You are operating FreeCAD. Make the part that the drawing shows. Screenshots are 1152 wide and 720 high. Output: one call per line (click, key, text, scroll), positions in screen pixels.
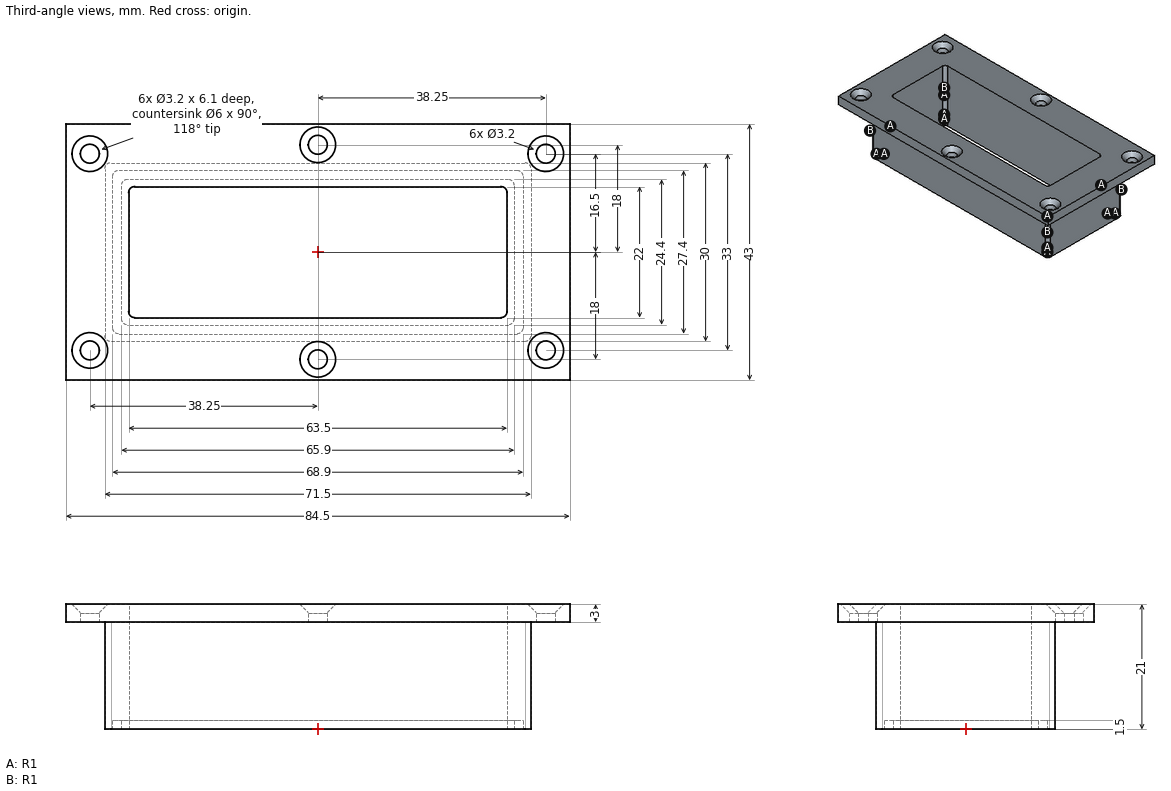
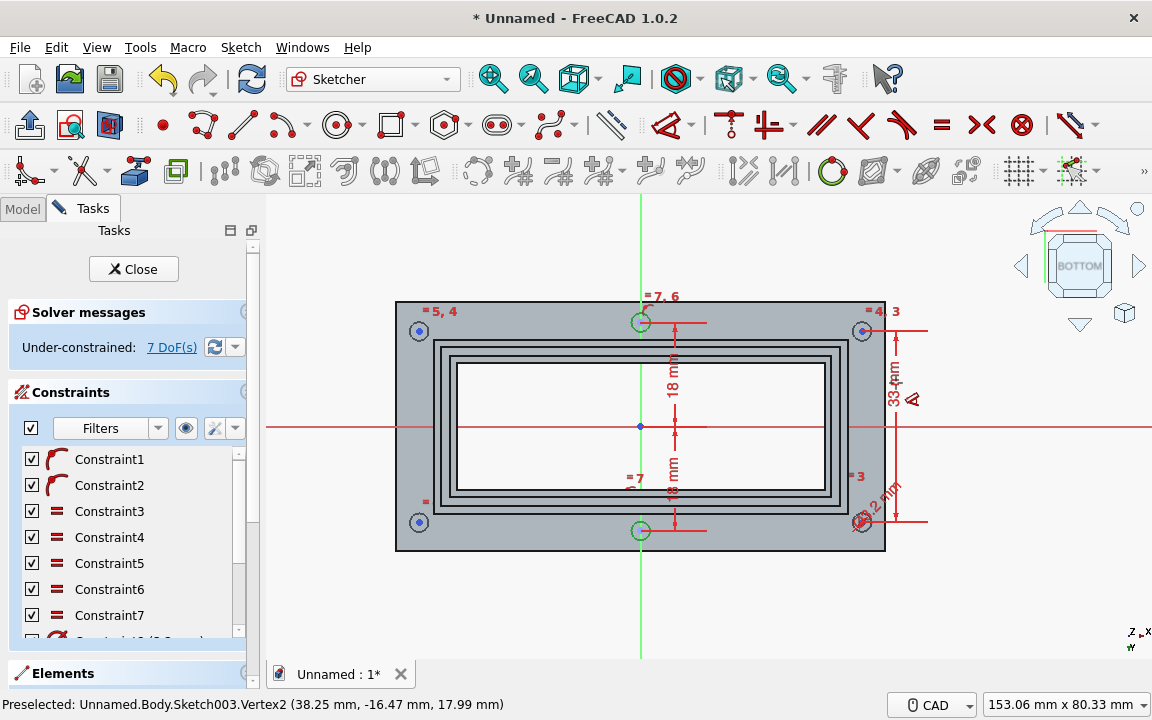
click(862, 522)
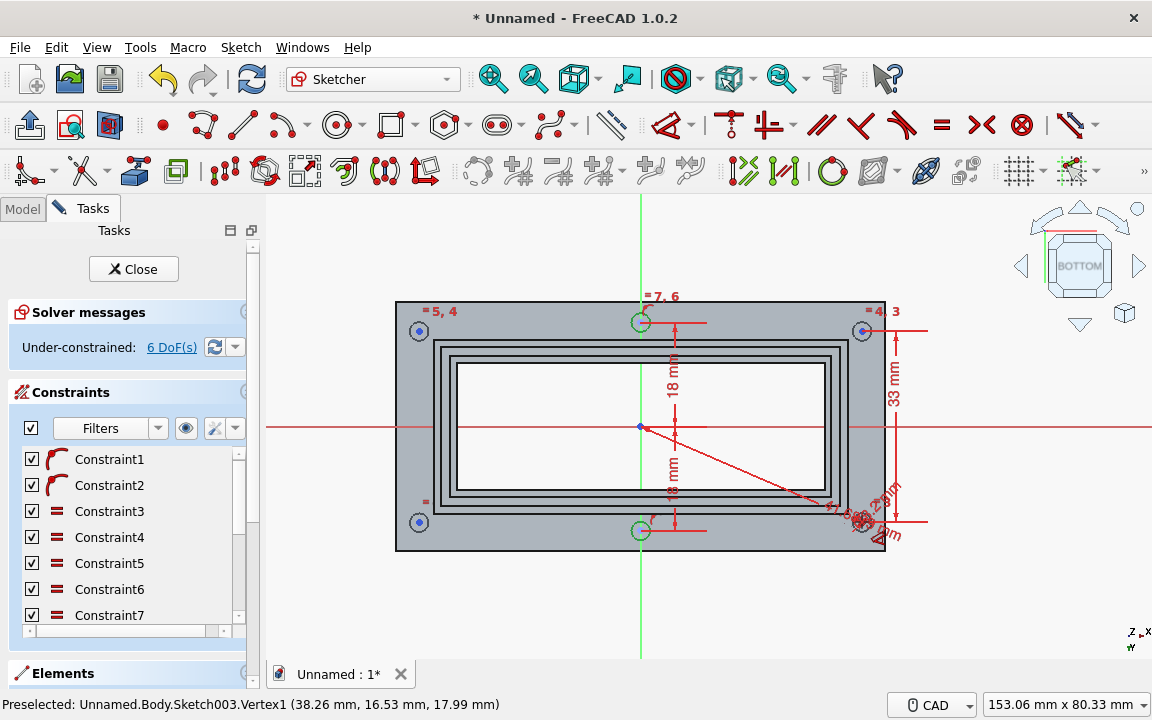
click(419, 331)
click(385, 383)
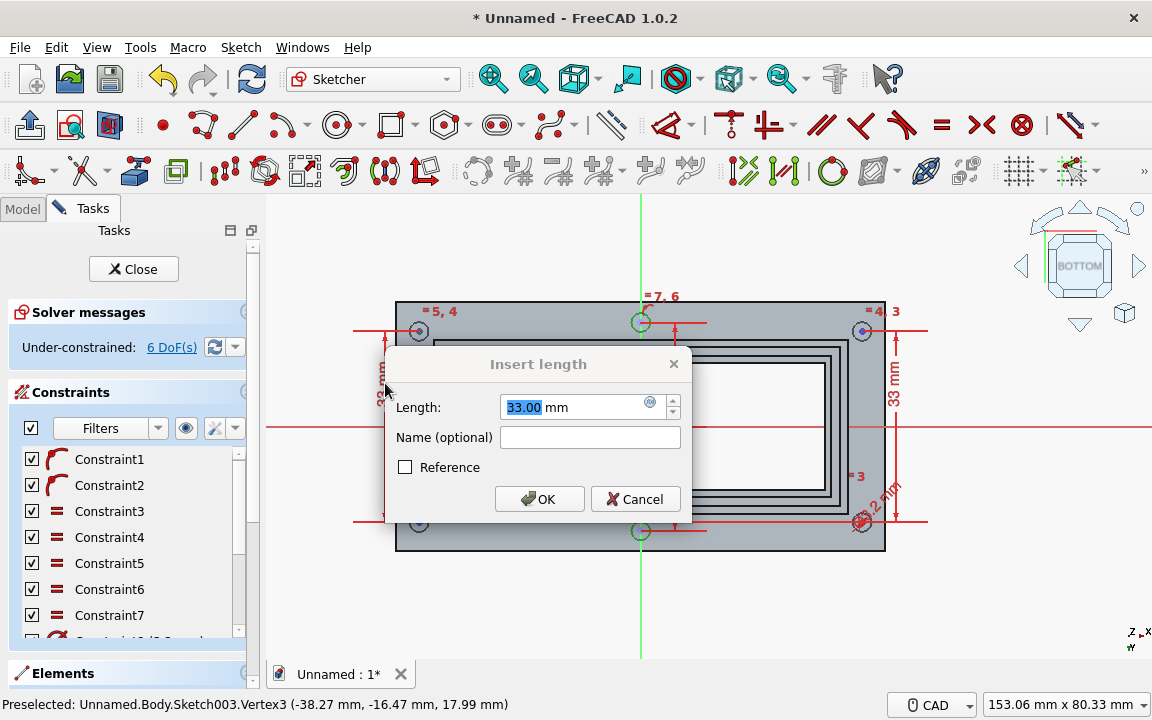
text(33)
key(Return)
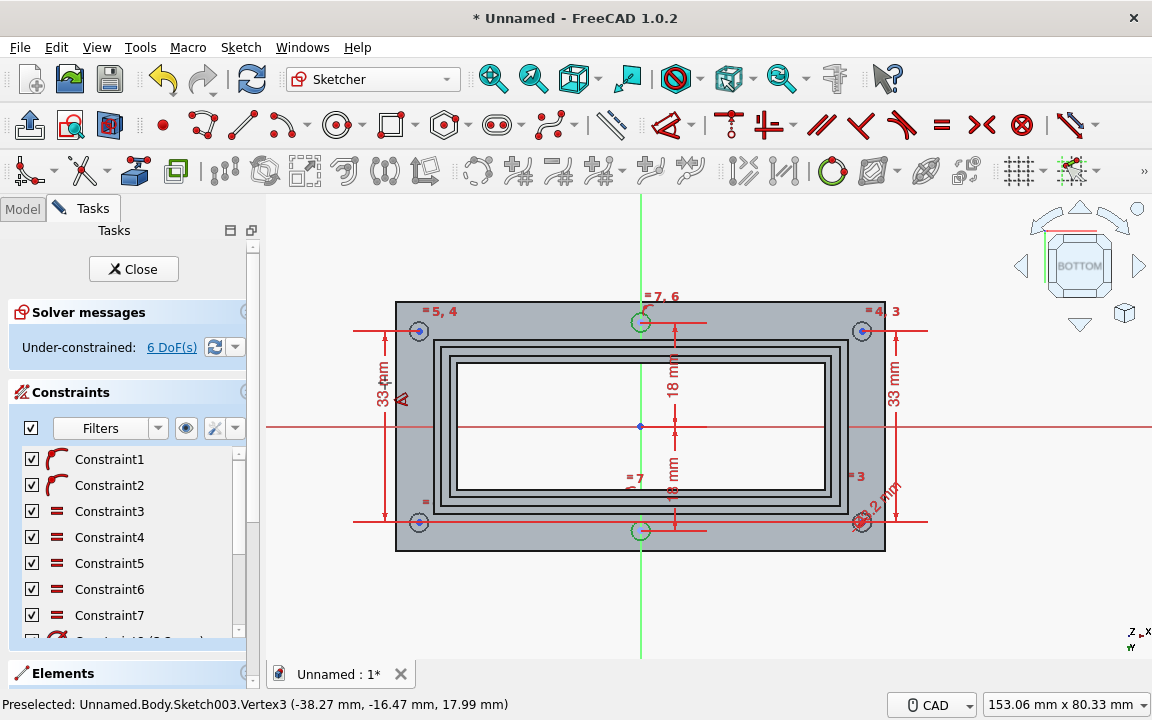
click(419, 331)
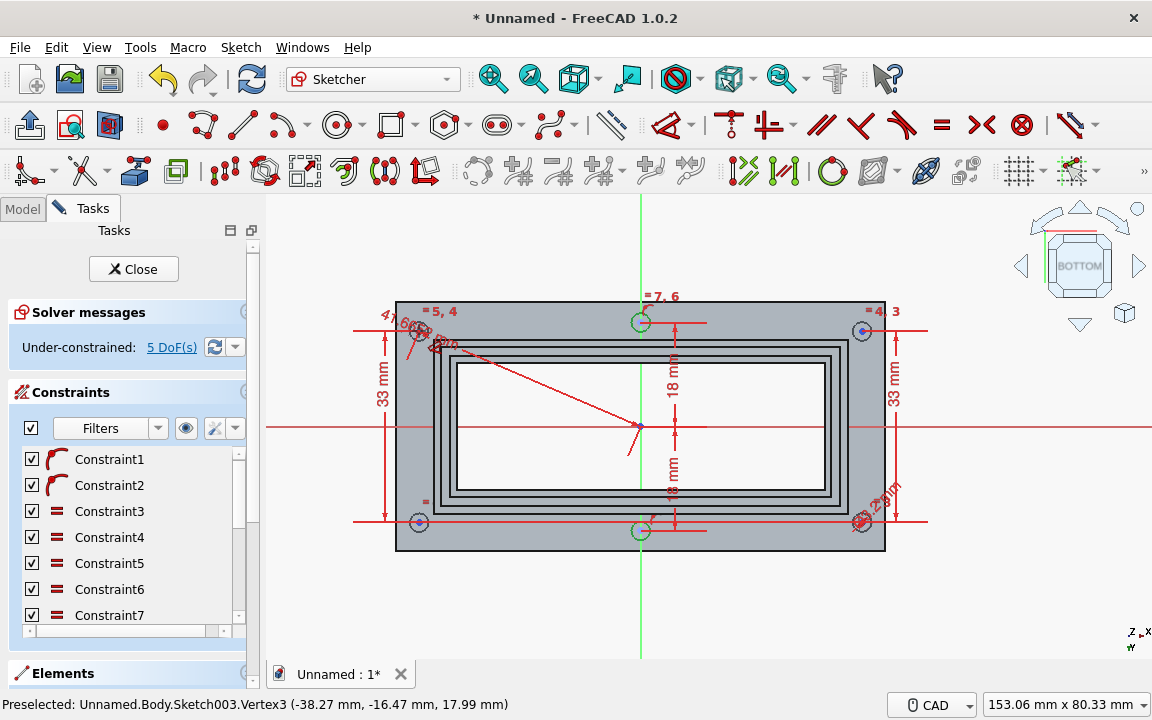
click(419, 523)
click(385, 471)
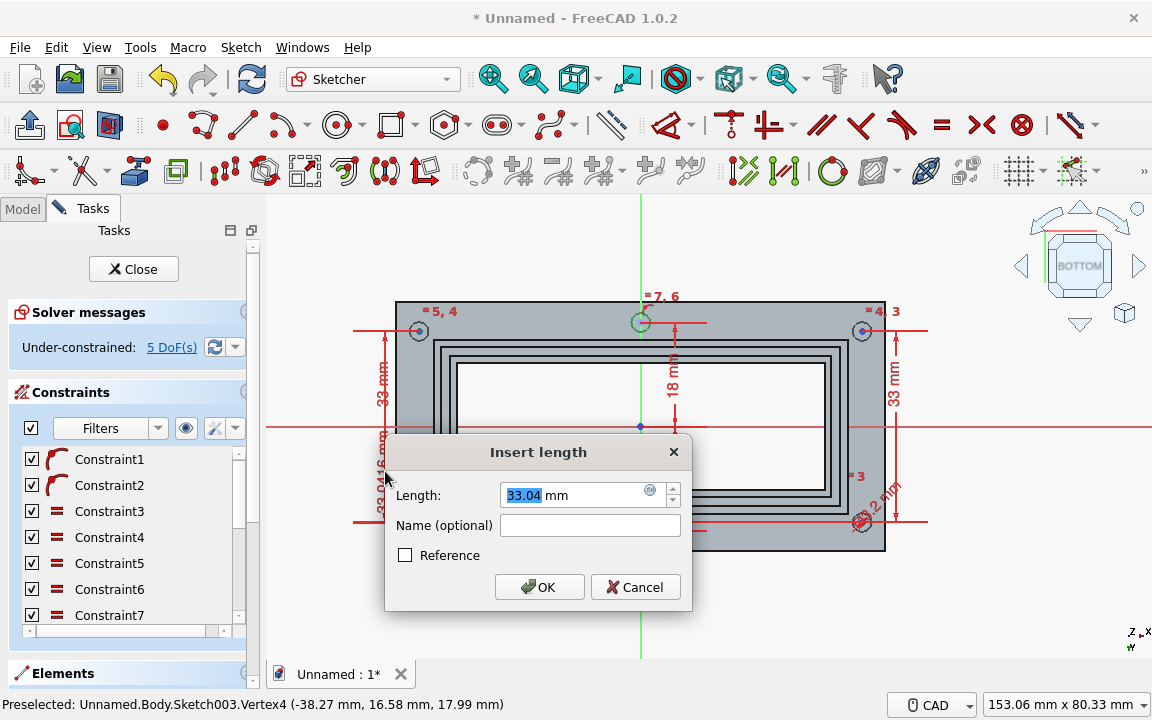
text(33)
key(Return)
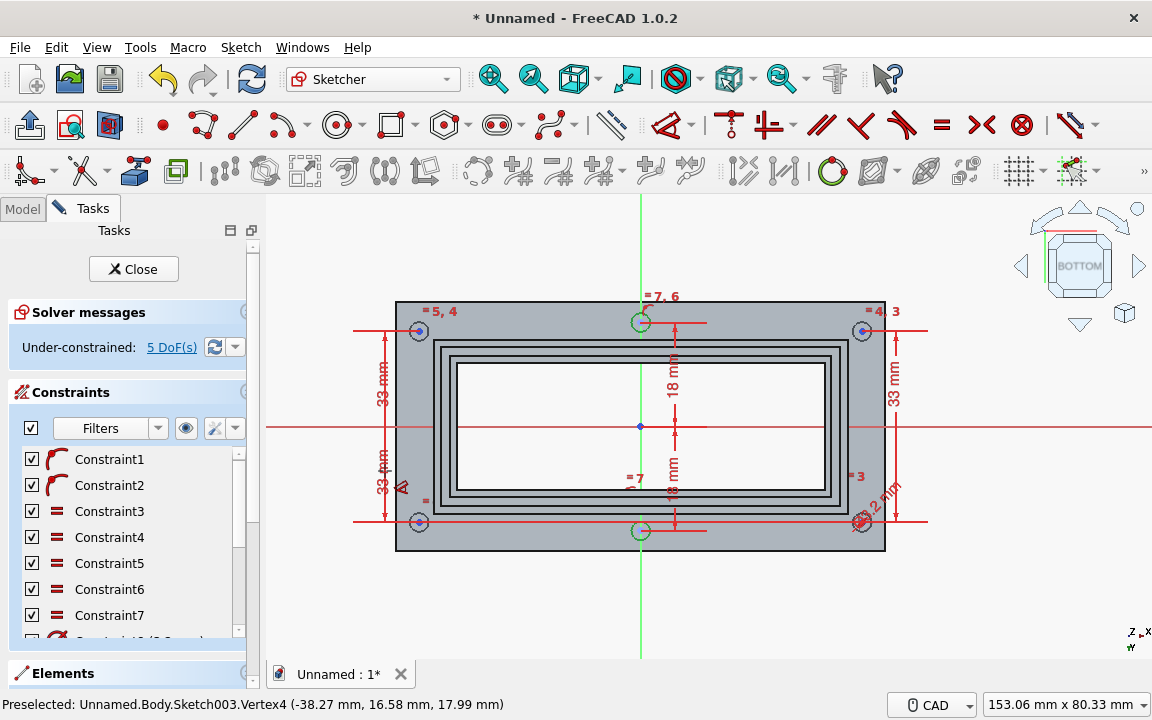
click(862, 522)
click(896, 475)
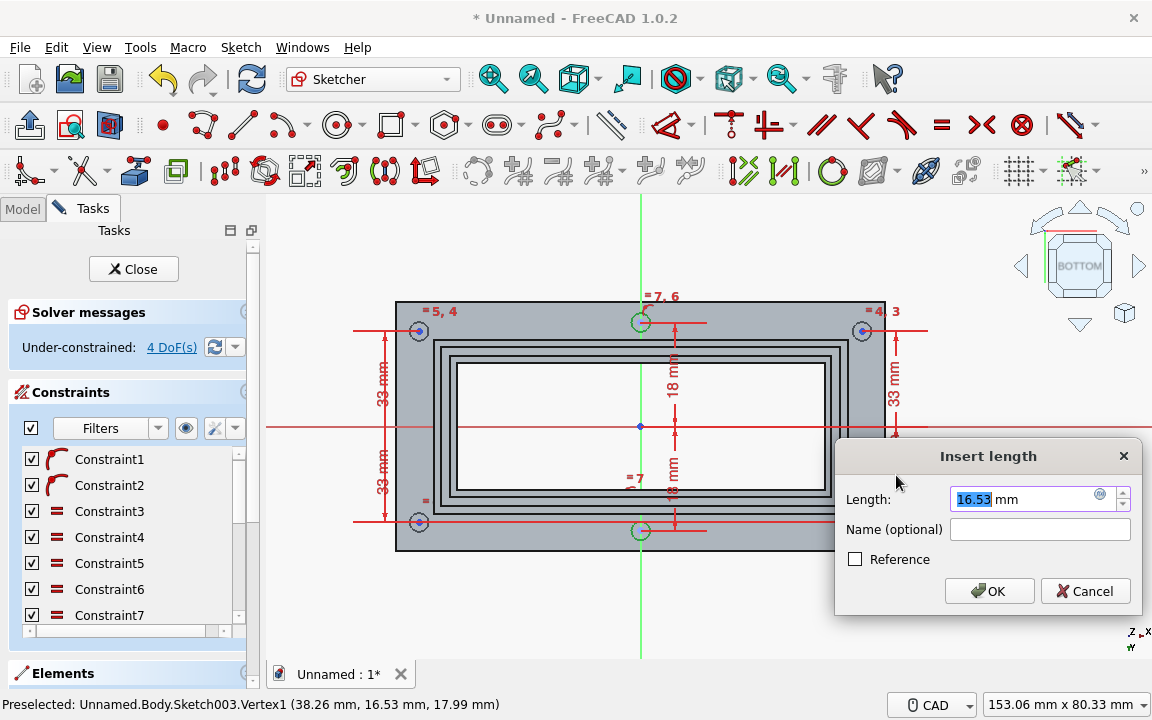
text(16.5)
key(Return)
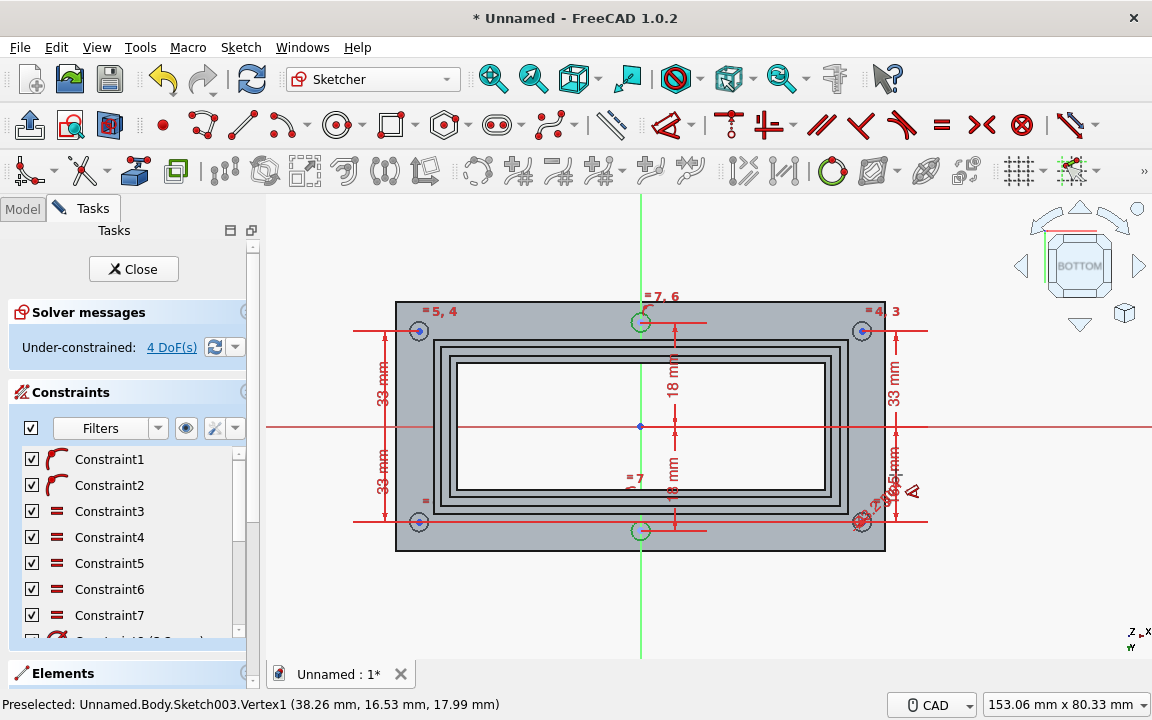
click(862, 522)
click(751, 556)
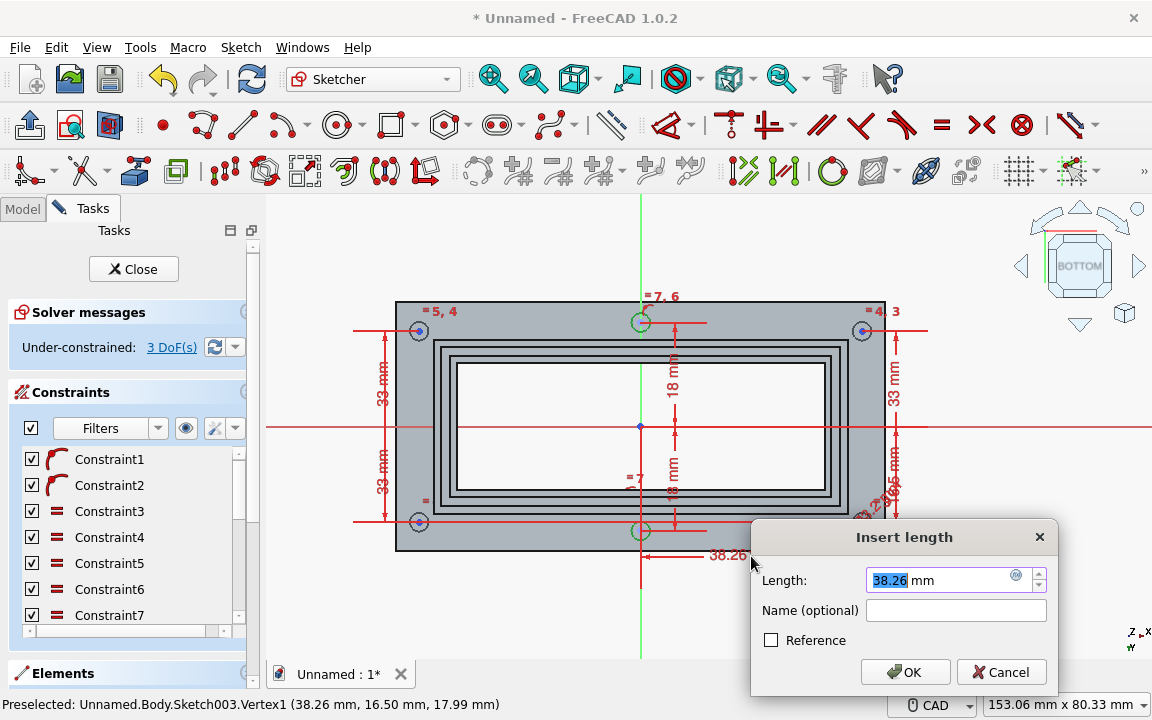
text(38.25)
key(Return)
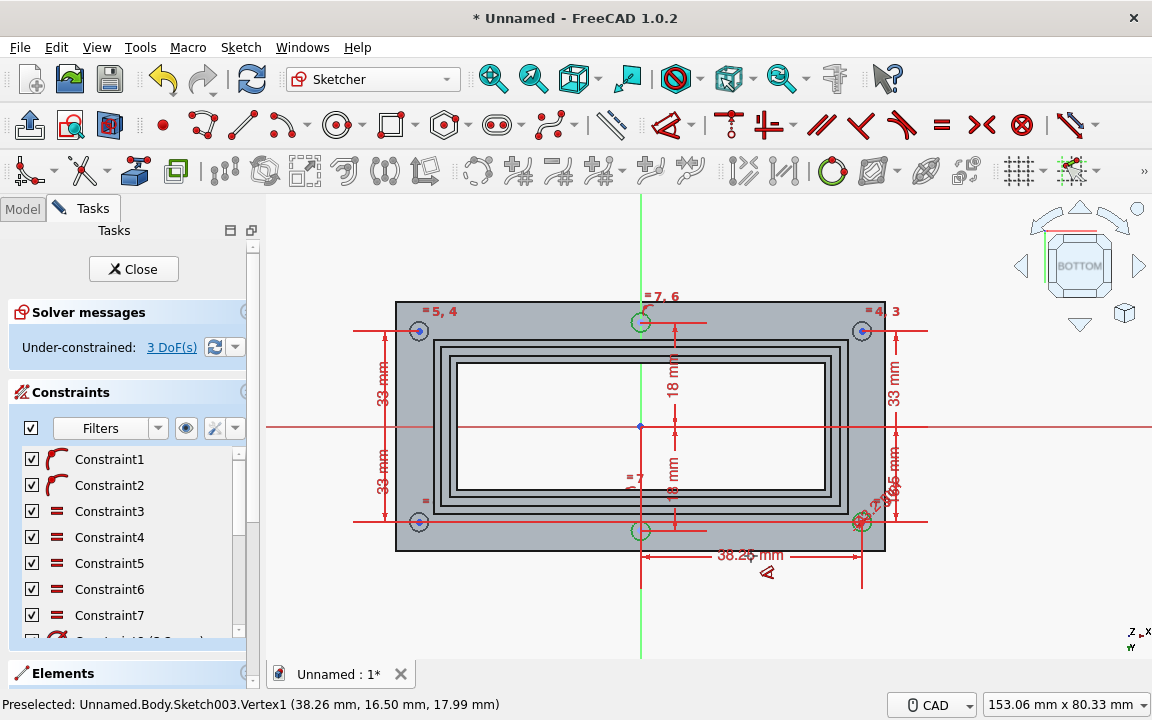
click(862, 331)
click(751, 297)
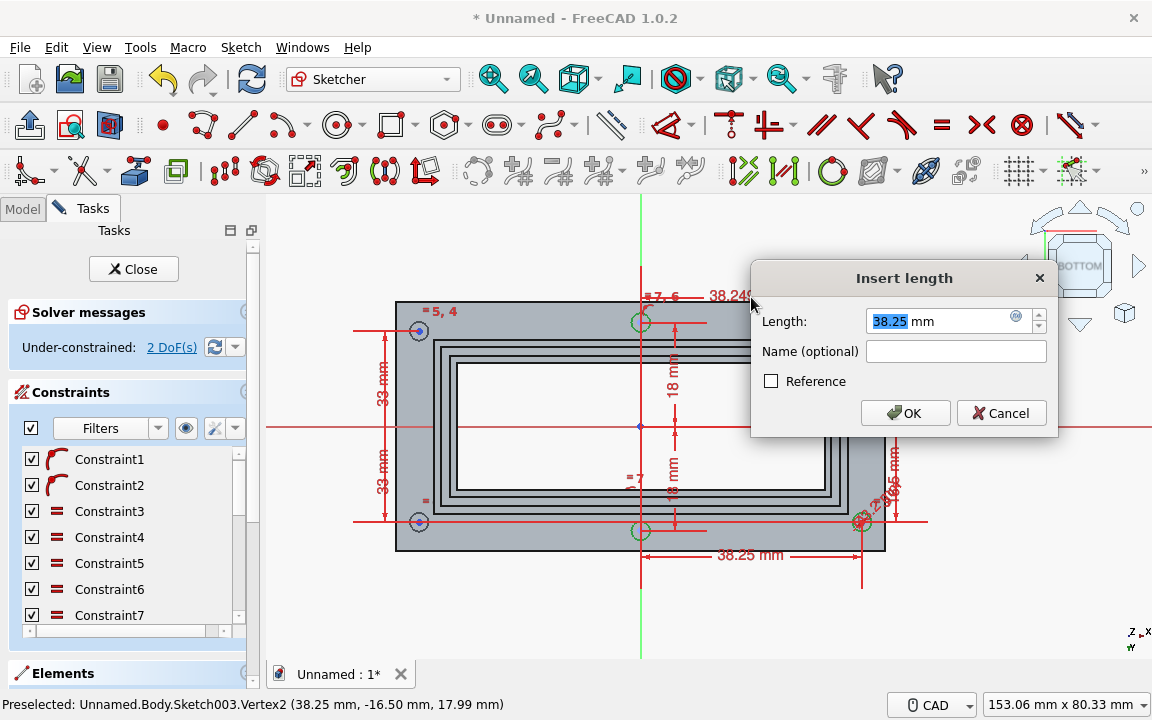
text(38.25)
key(Return)